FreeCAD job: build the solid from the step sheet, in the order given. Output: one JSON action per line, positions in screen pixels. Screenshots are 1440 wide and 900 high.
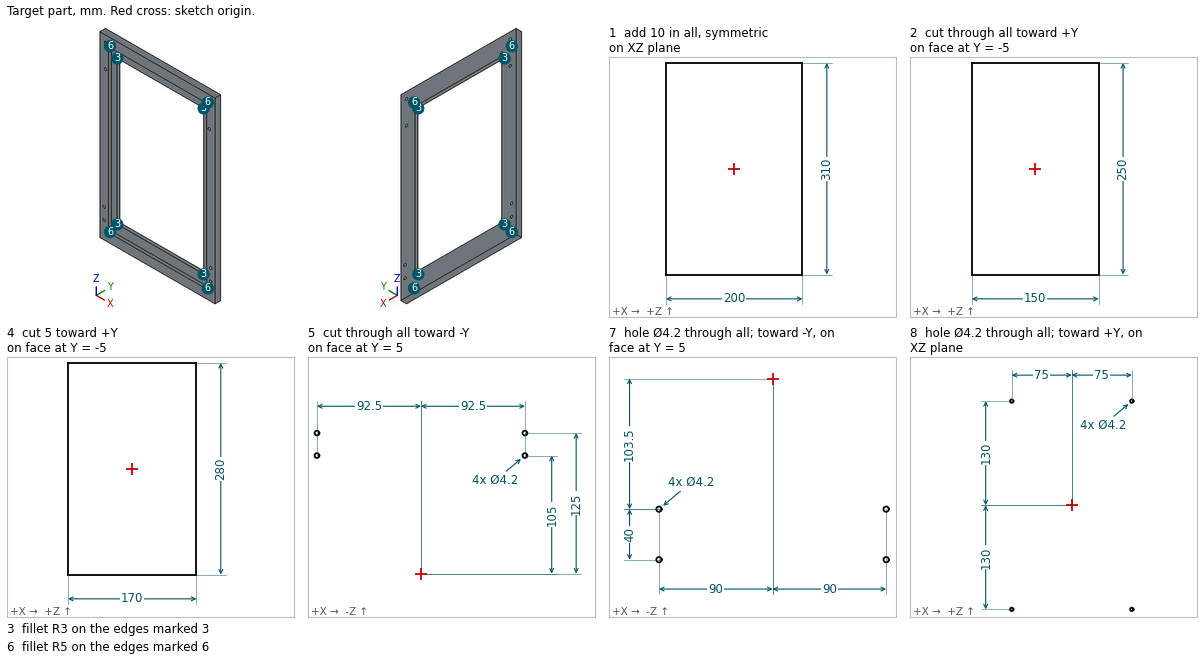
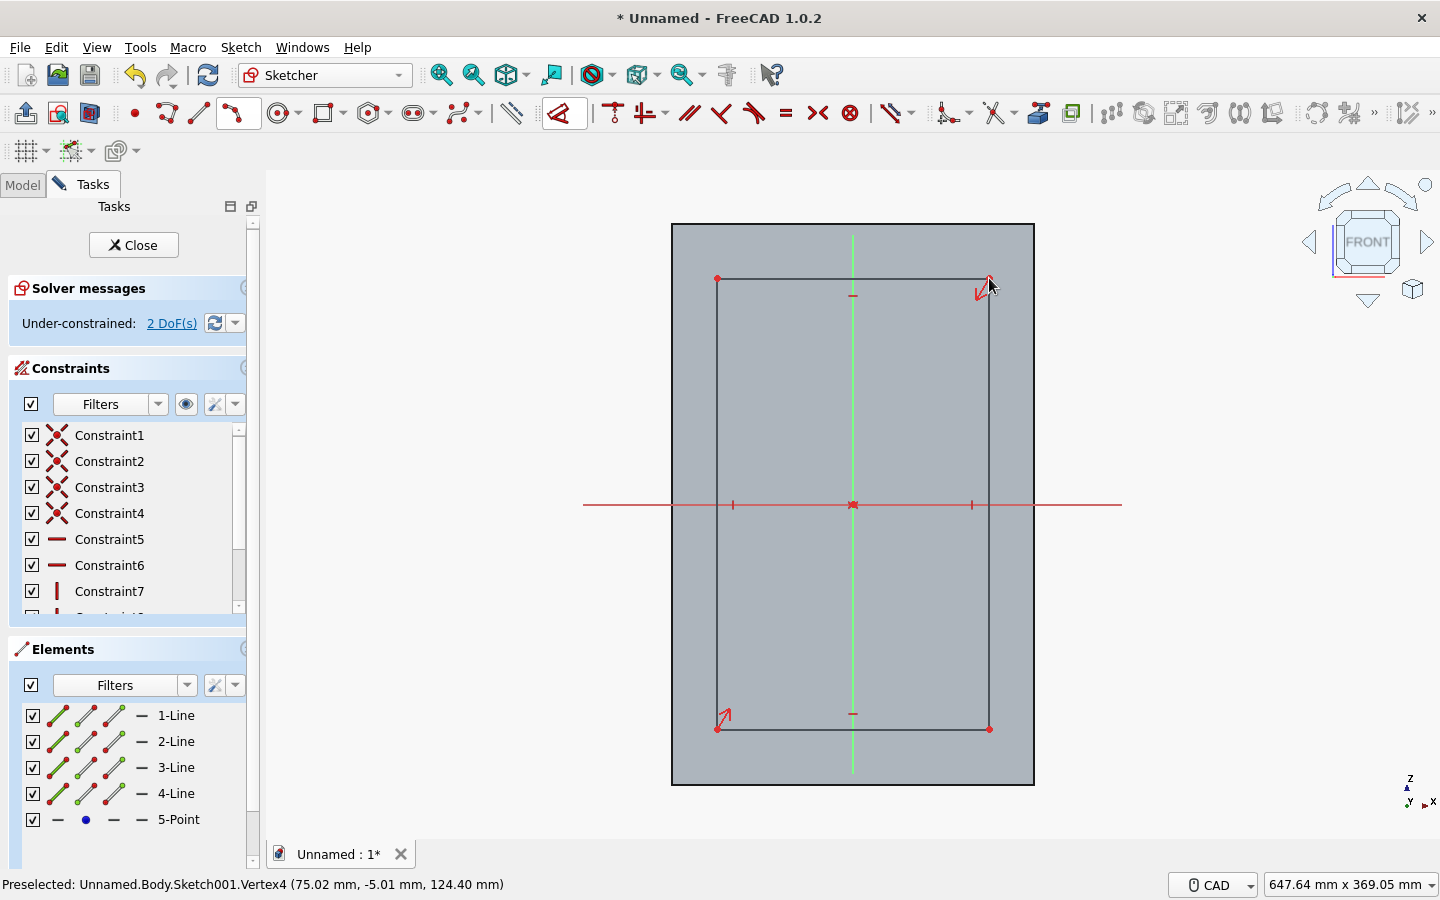
{"action": "left_click", "coordinate": [799, 730]}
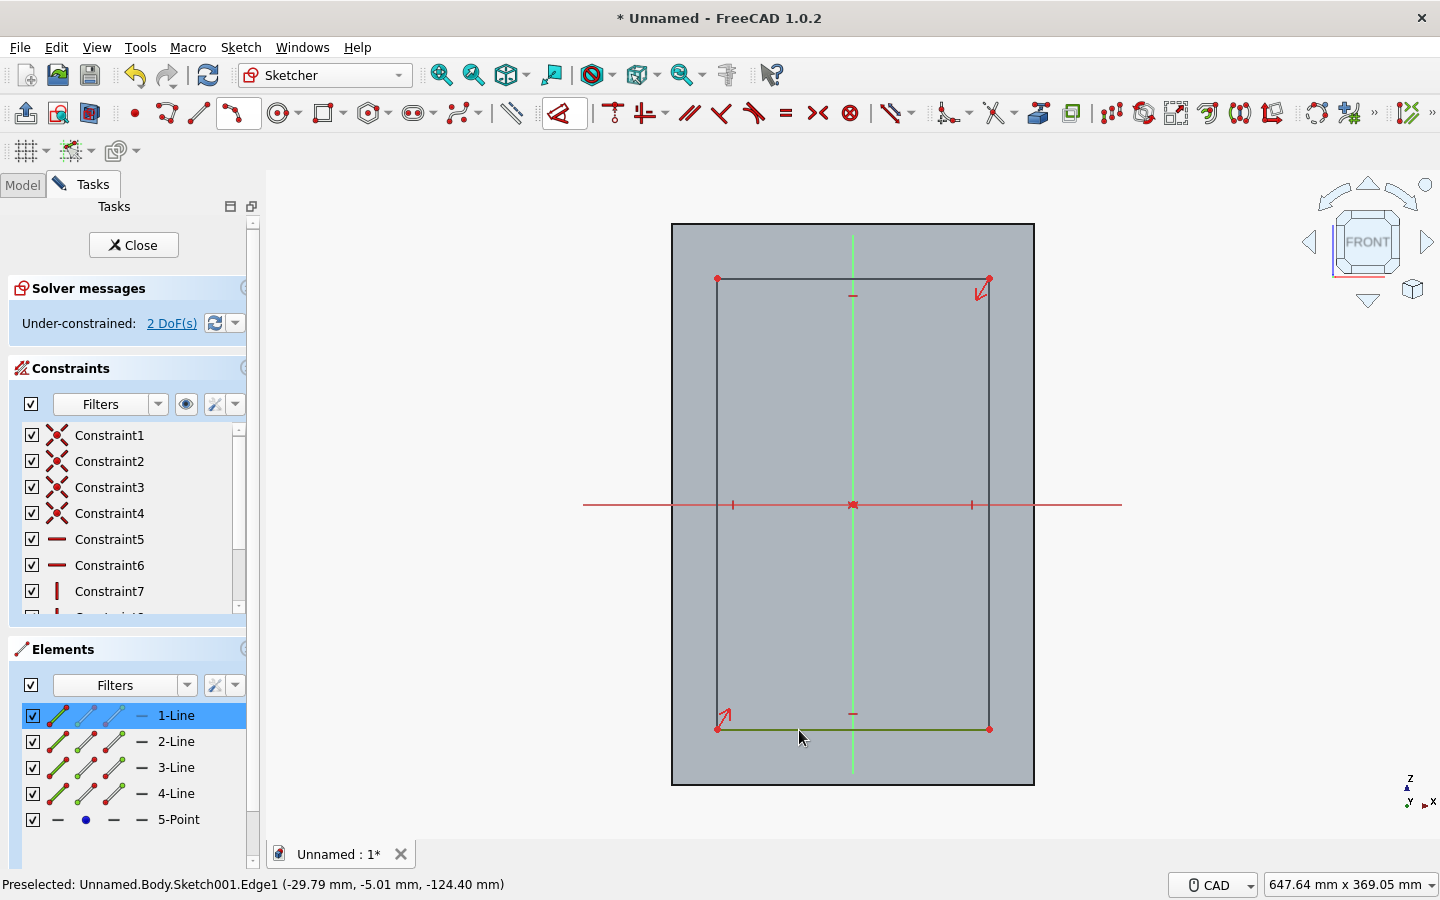
{"action": "left_click", "coordinate": [582, 114]}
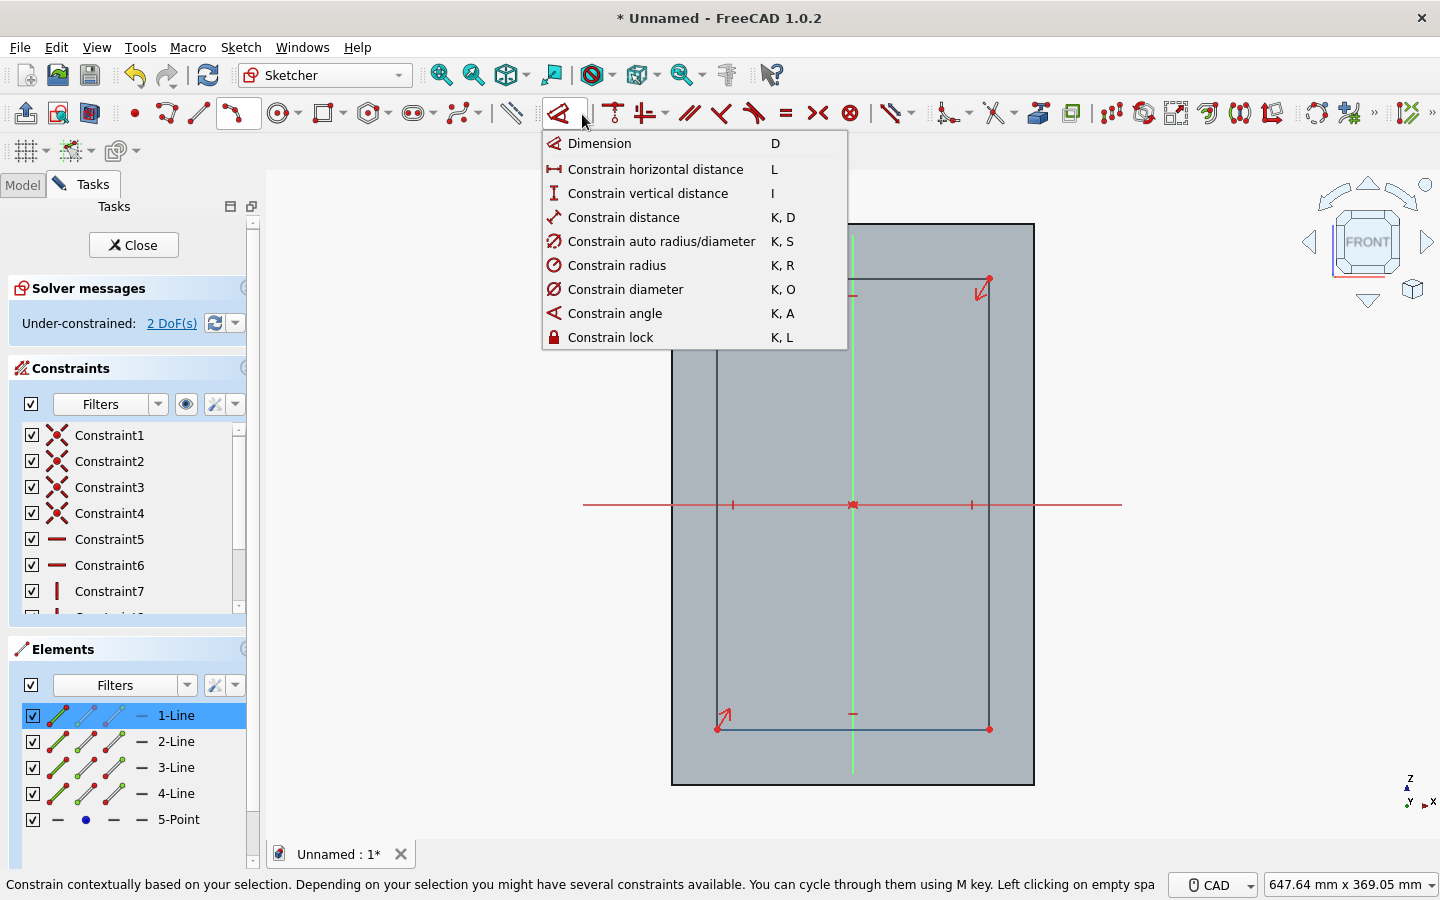
{"action": "left_click", "coordinate": [695, 169]}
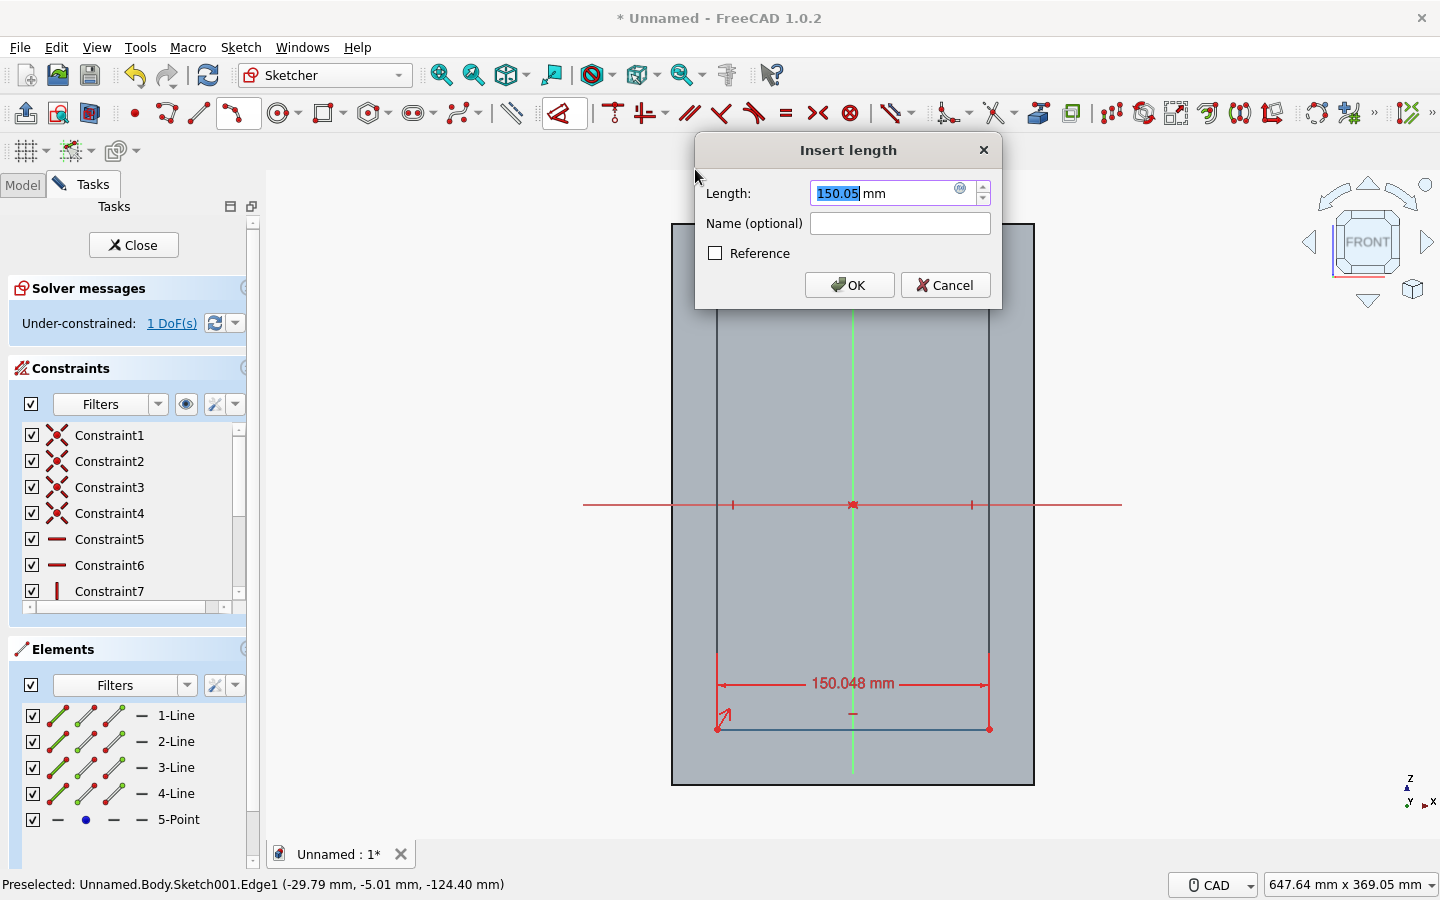
{"action": "type", "text": "150"}
{"action": "key", "text": "Return"}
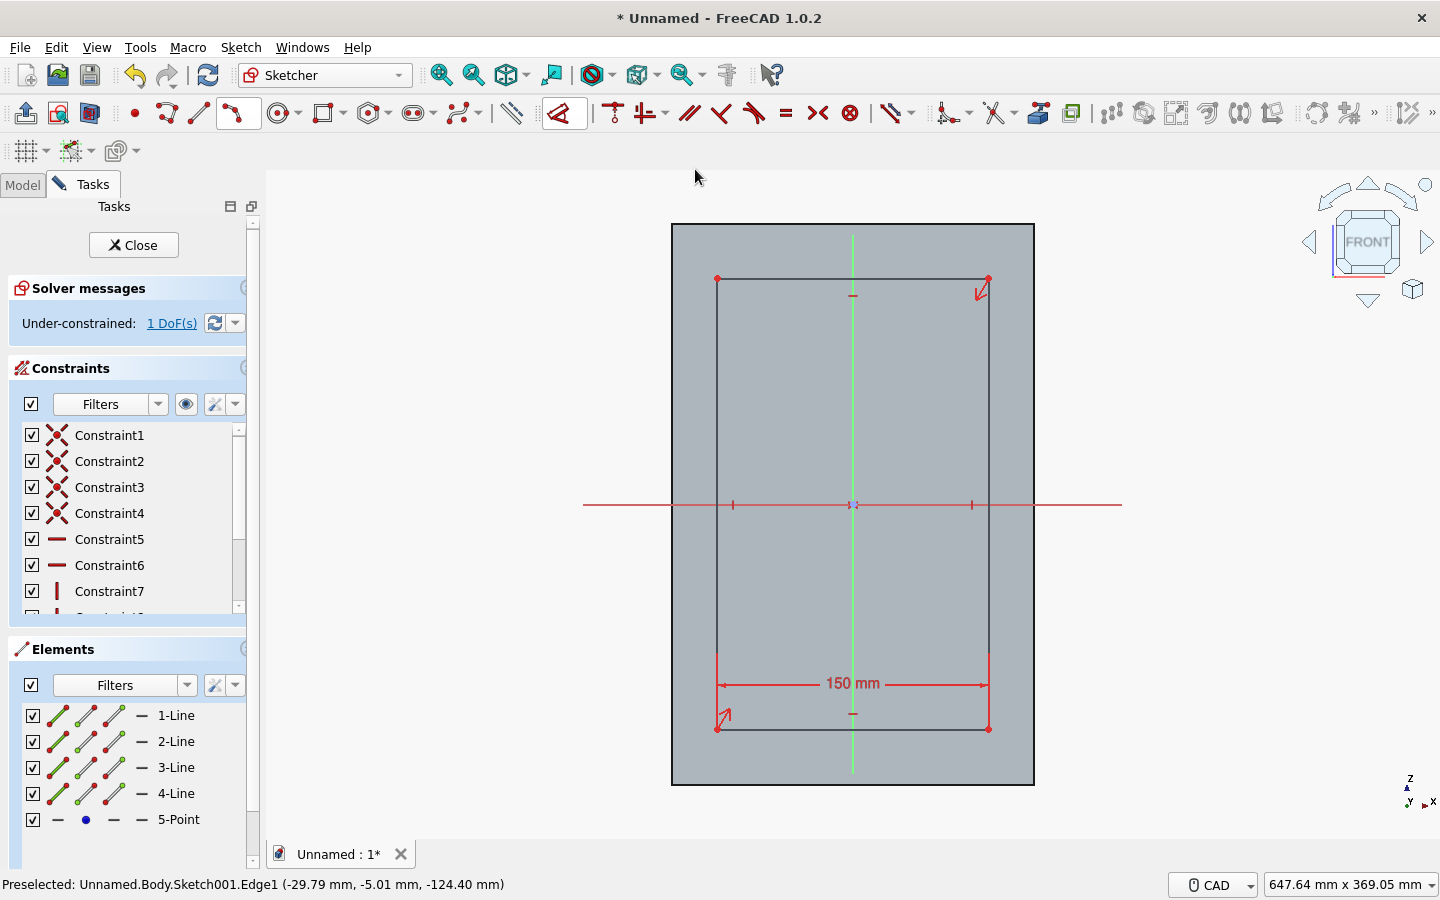
{"action": "left_click", "coordinate": [989, 595]}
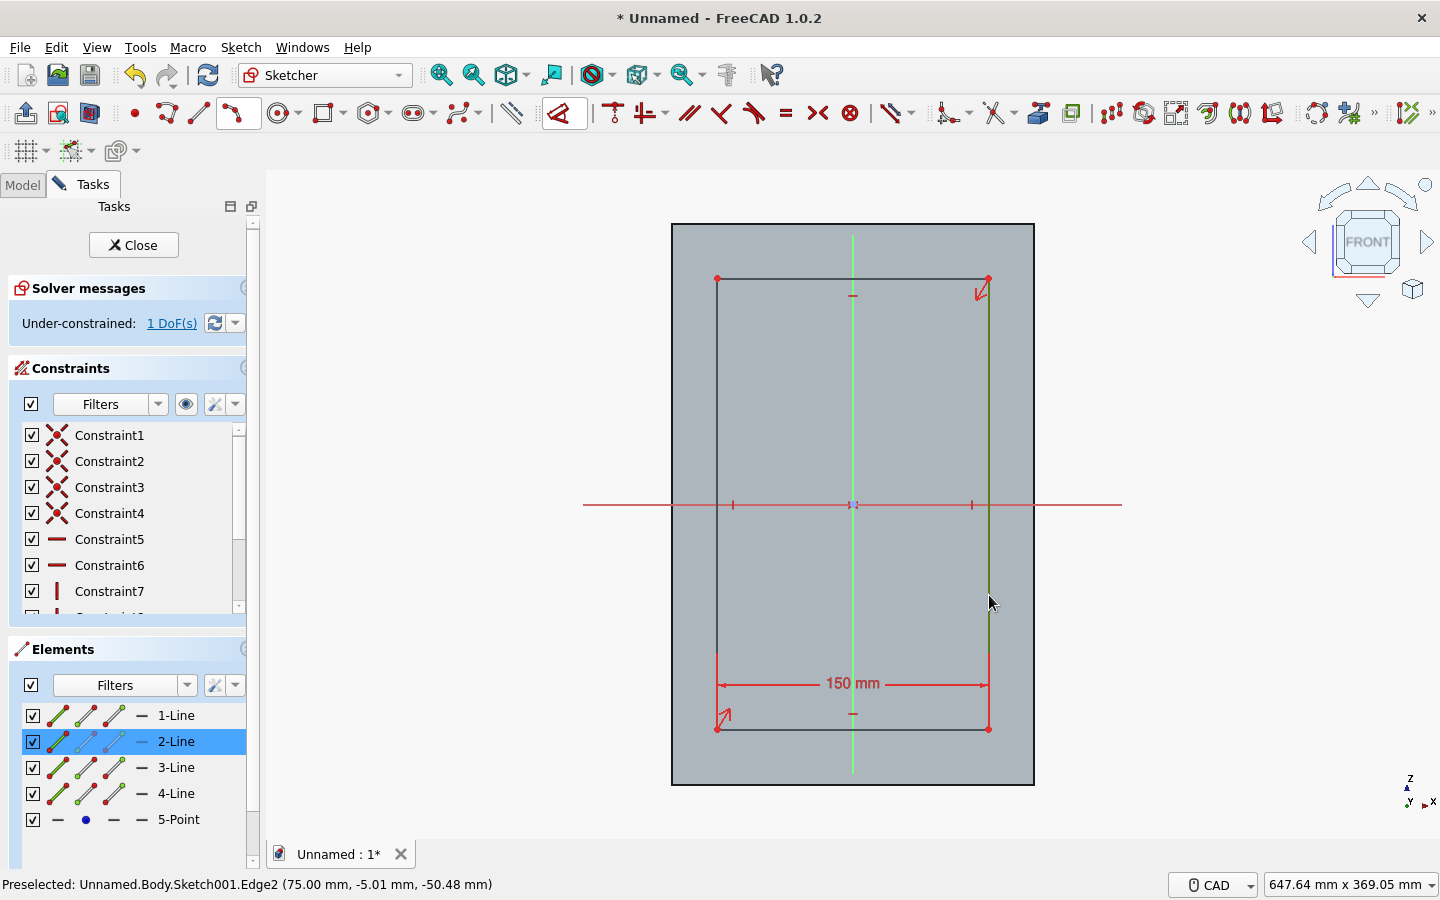
{"action": "key", "text": "i"}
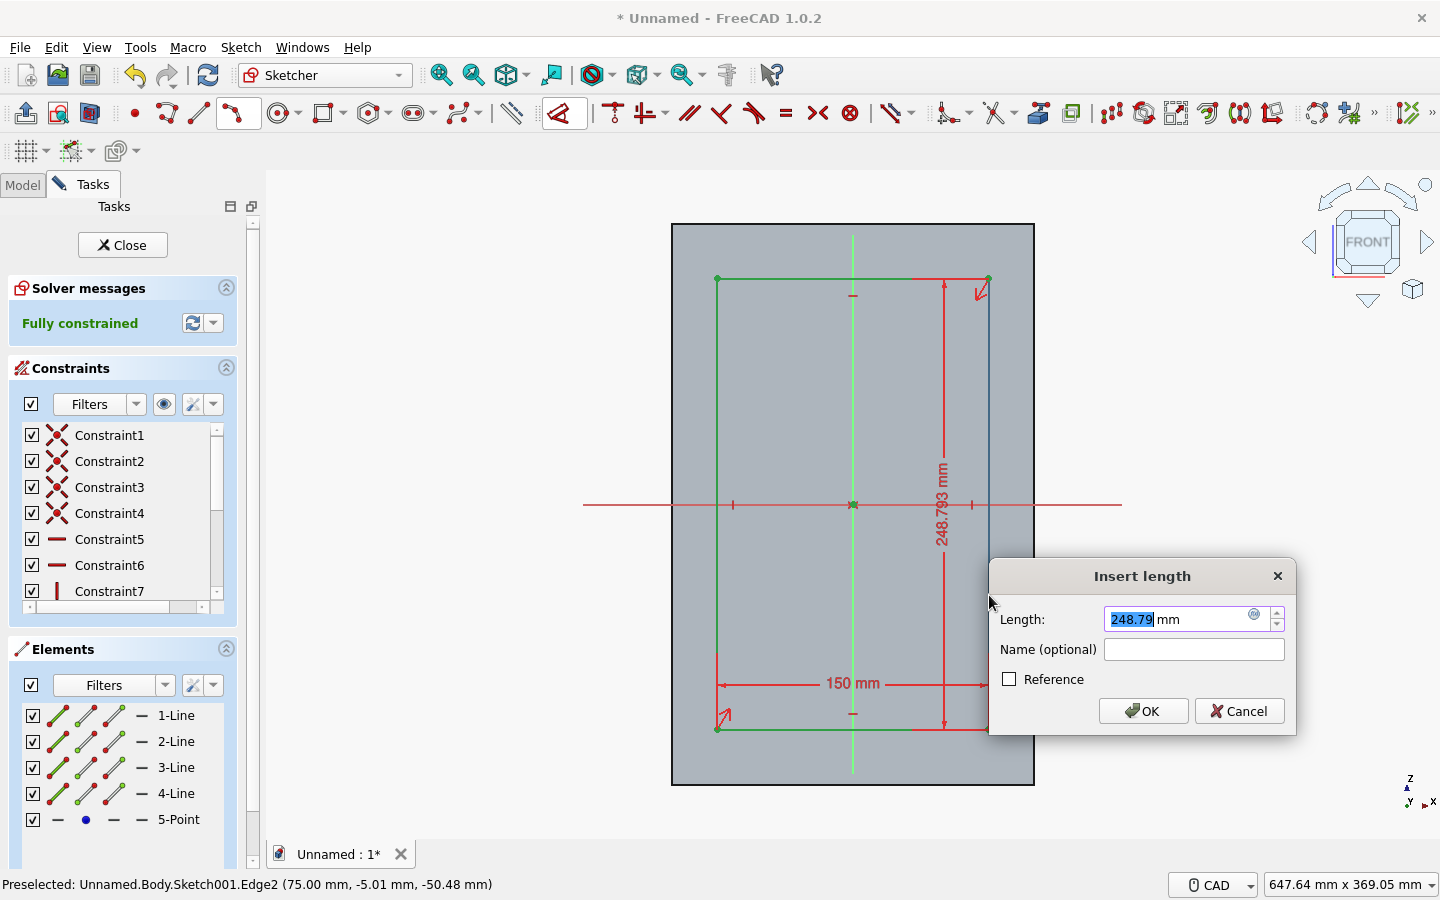
{"action": "type", "text": "250"}
{"action": "key", "text": "Return"}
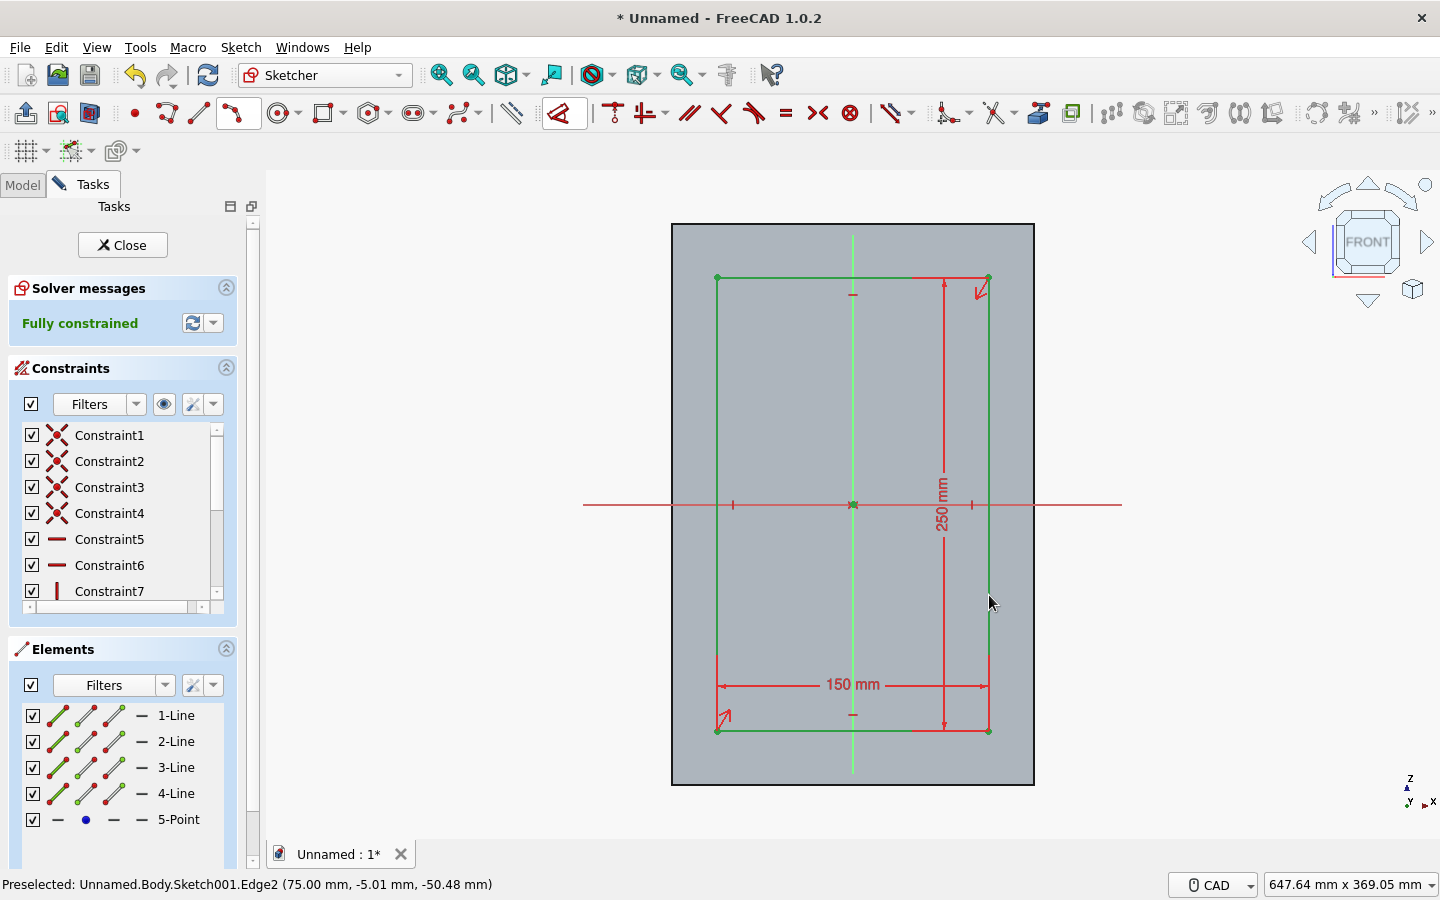
{"action": "left_click", "coordinate": [123, 245]}